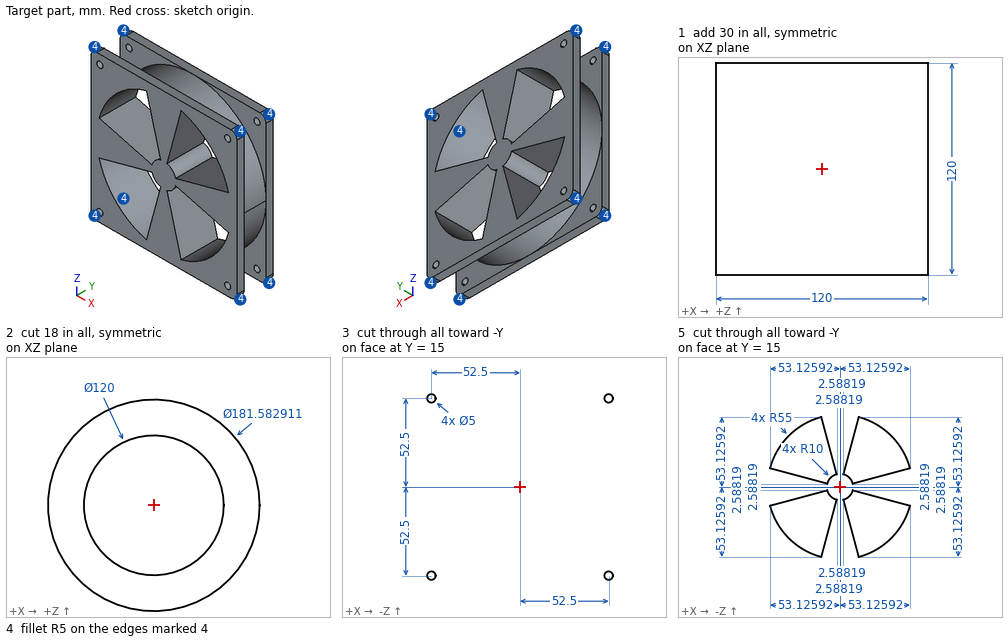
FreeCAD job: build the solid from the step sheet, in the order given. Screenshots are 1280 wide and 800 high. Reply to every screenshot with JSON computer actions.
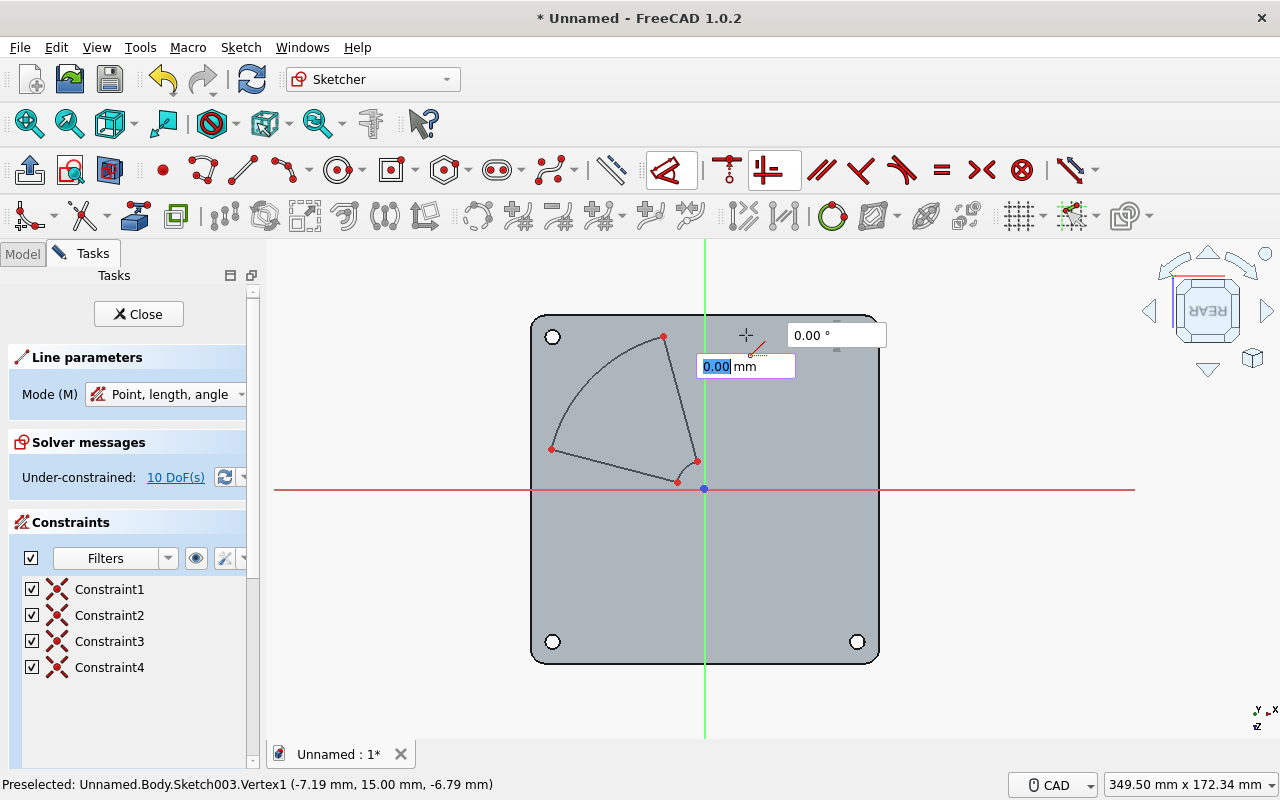
{"action": "scroll", "coordinate": [712, 462], "scroll_direction": "up", "scroll_amount": 4}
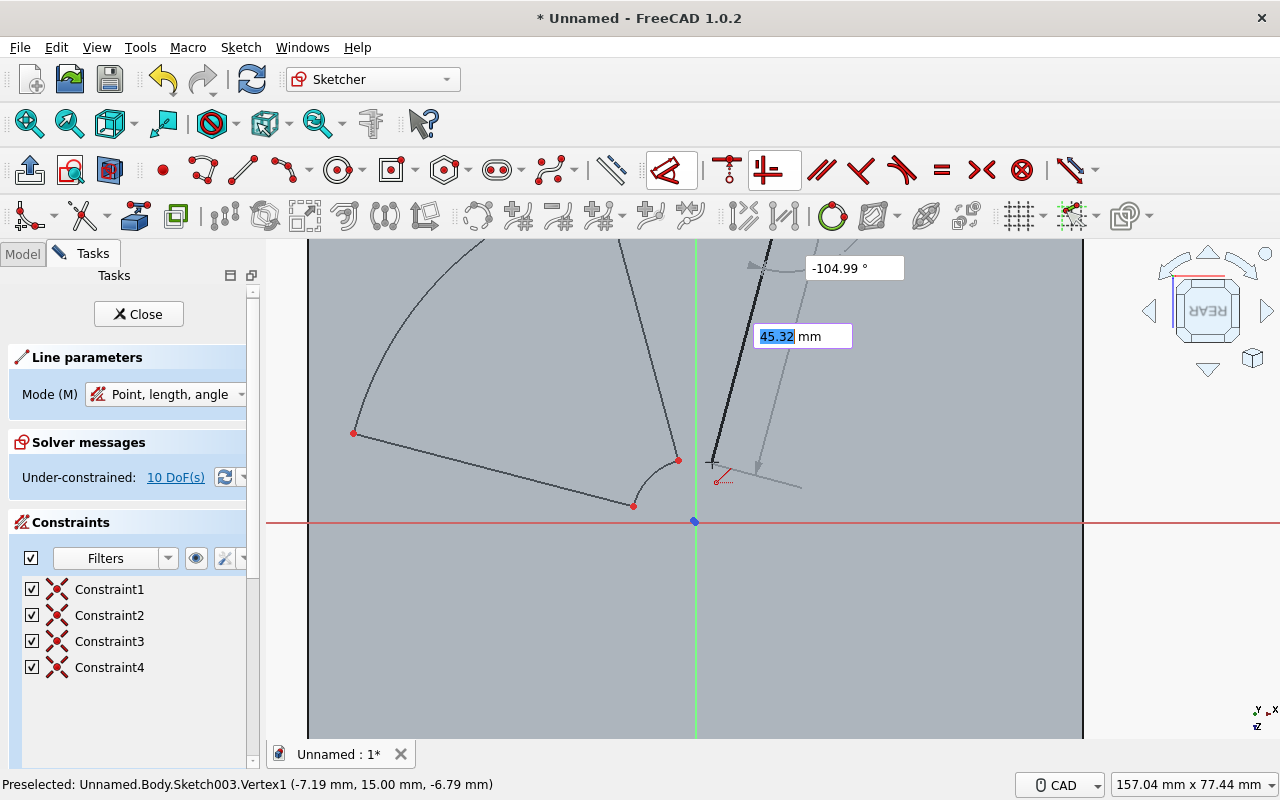
{"action": "left_click", "coordinate": [712, 460]}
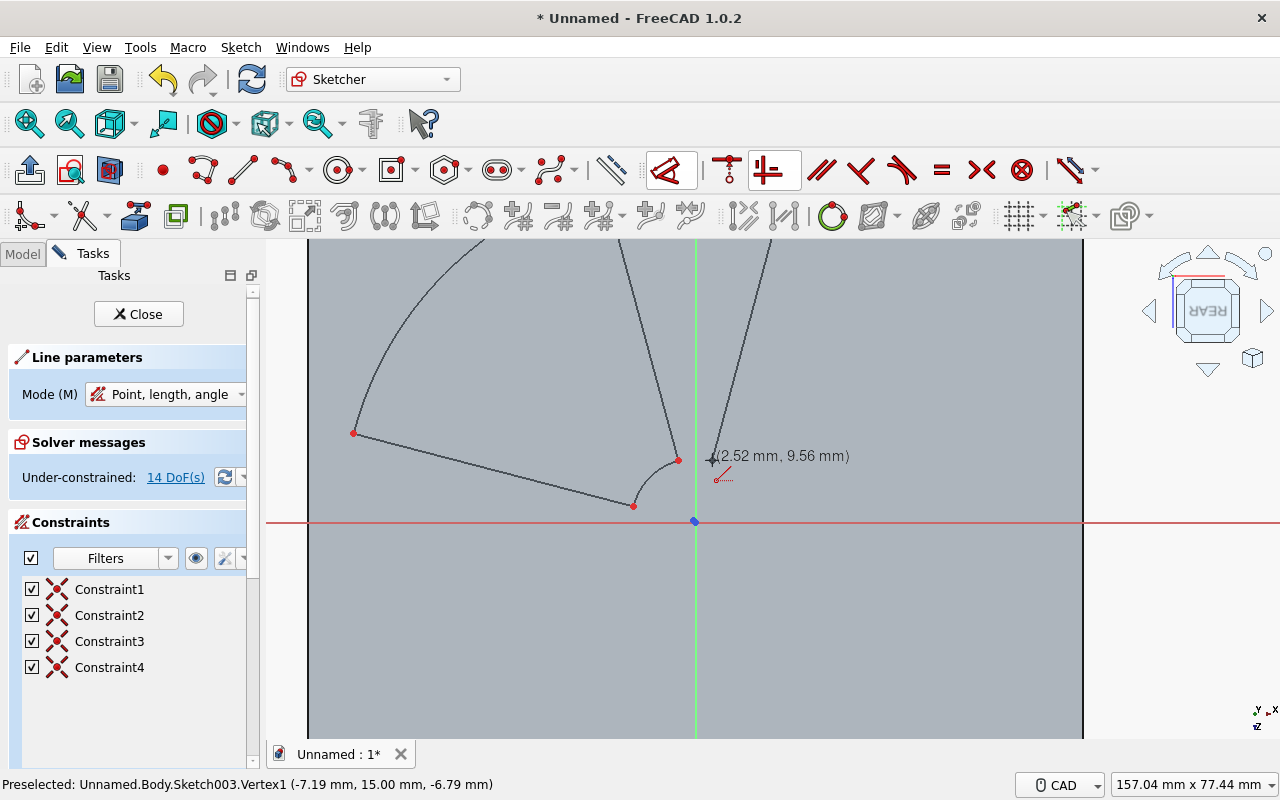
{"action": "left_click", "coordinate": [758, 506]}
{"action": "left_click", "coordinate": [1039, 431]}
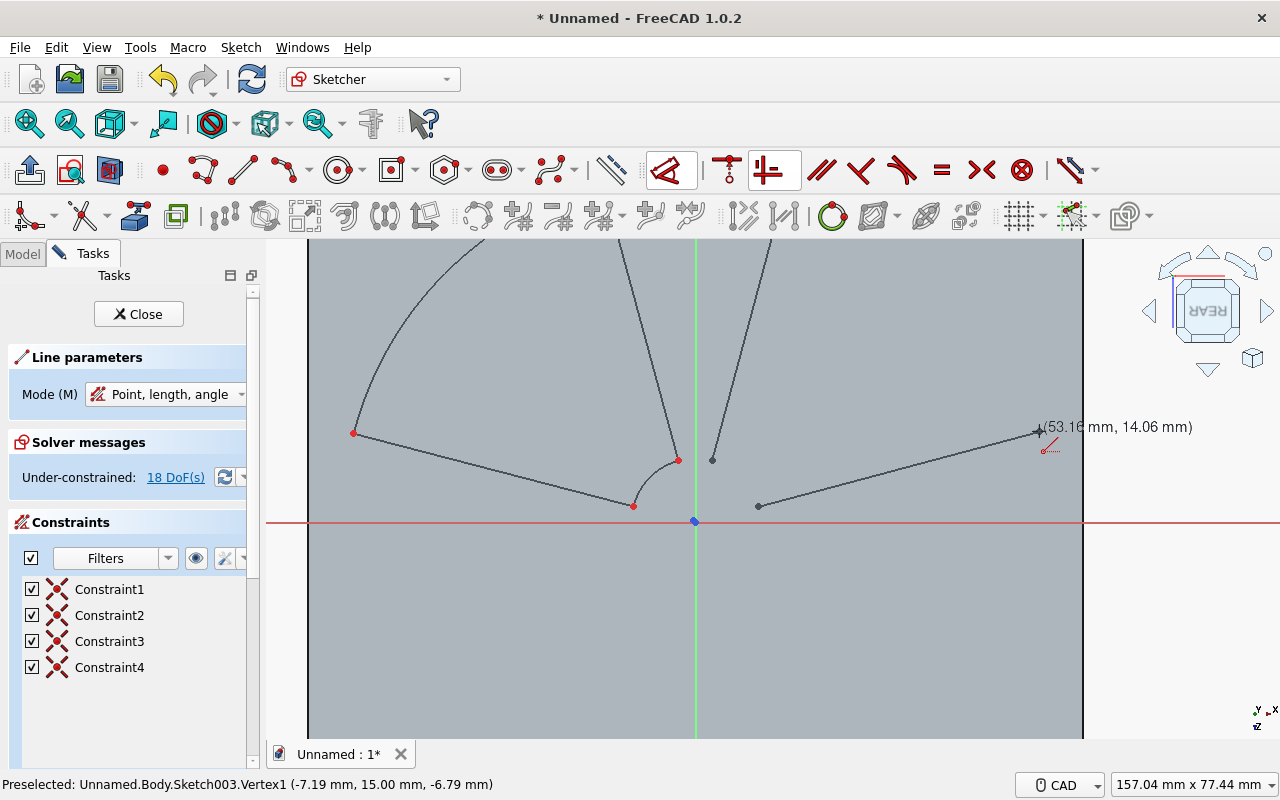
{"action": "left_click", "coordinate": [284, 170]}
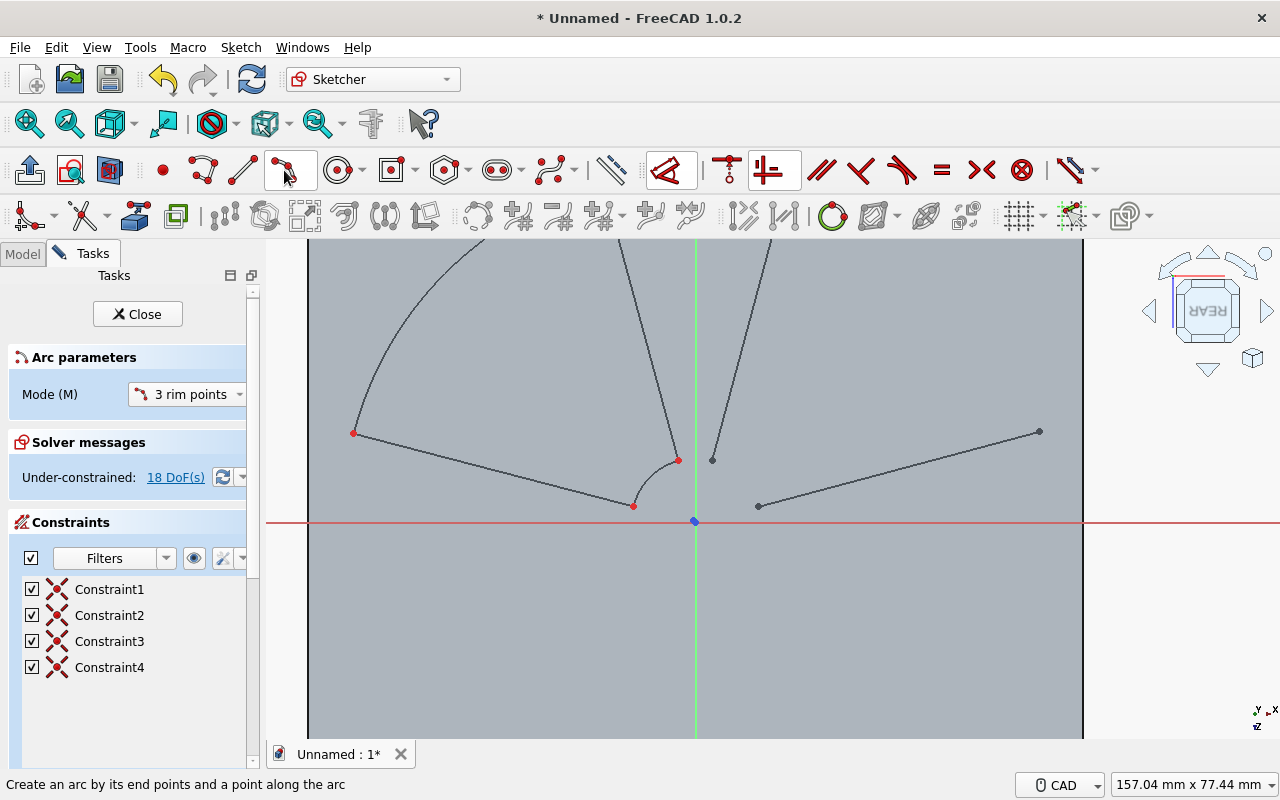
{"action": "left_click", "coordinate": [712, 461]}
{"action": "left_click", "coordinate": [758, 507]}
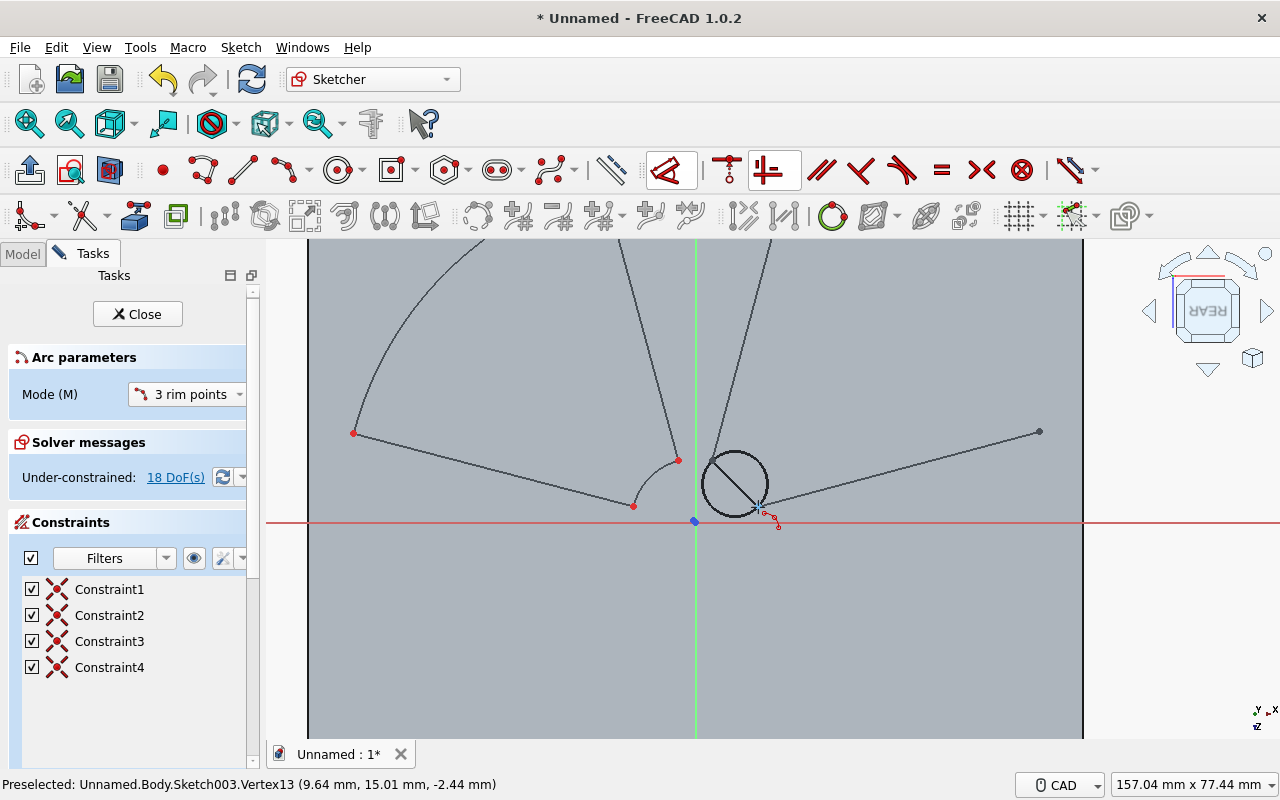
{"action": "scroll", "coordinate": [741, 477], "scroll_direction": "up", "scroll_amount": 4}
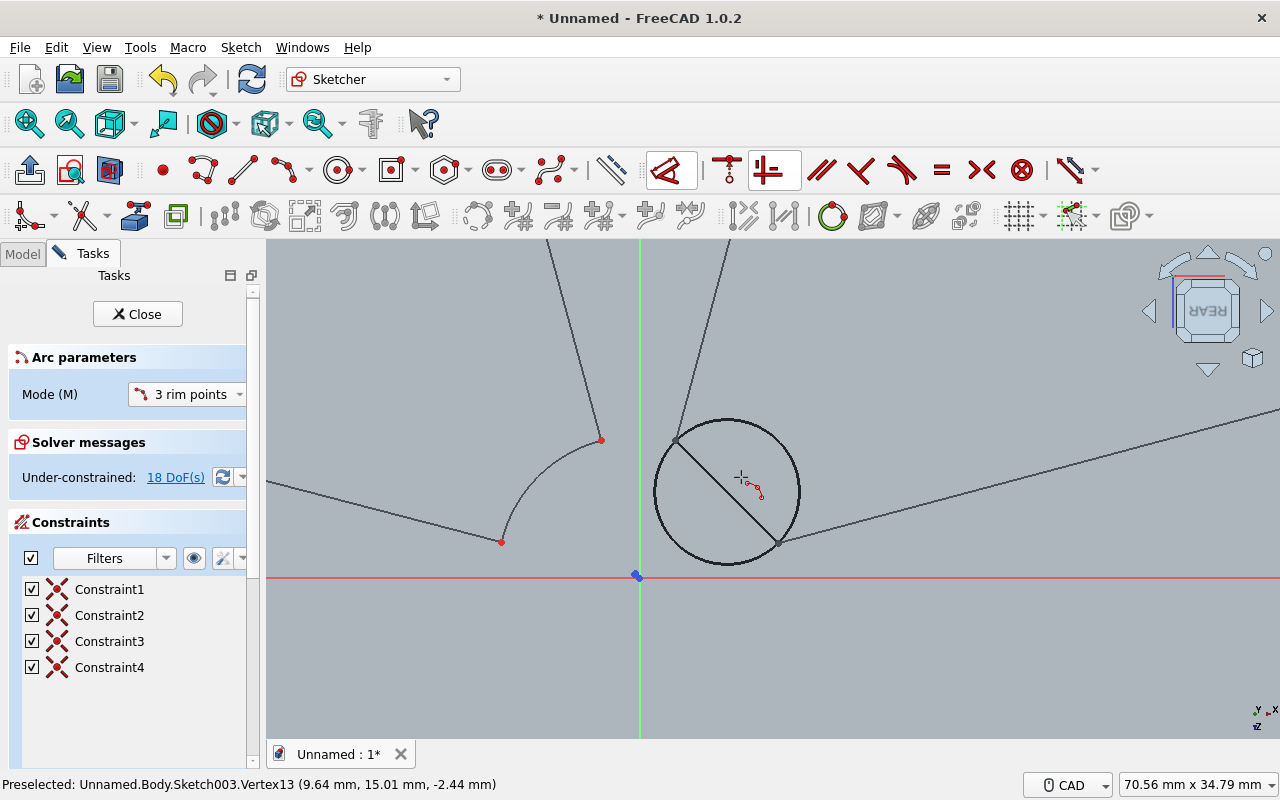
{"action": "left_click", "coordinate": [741, 477]}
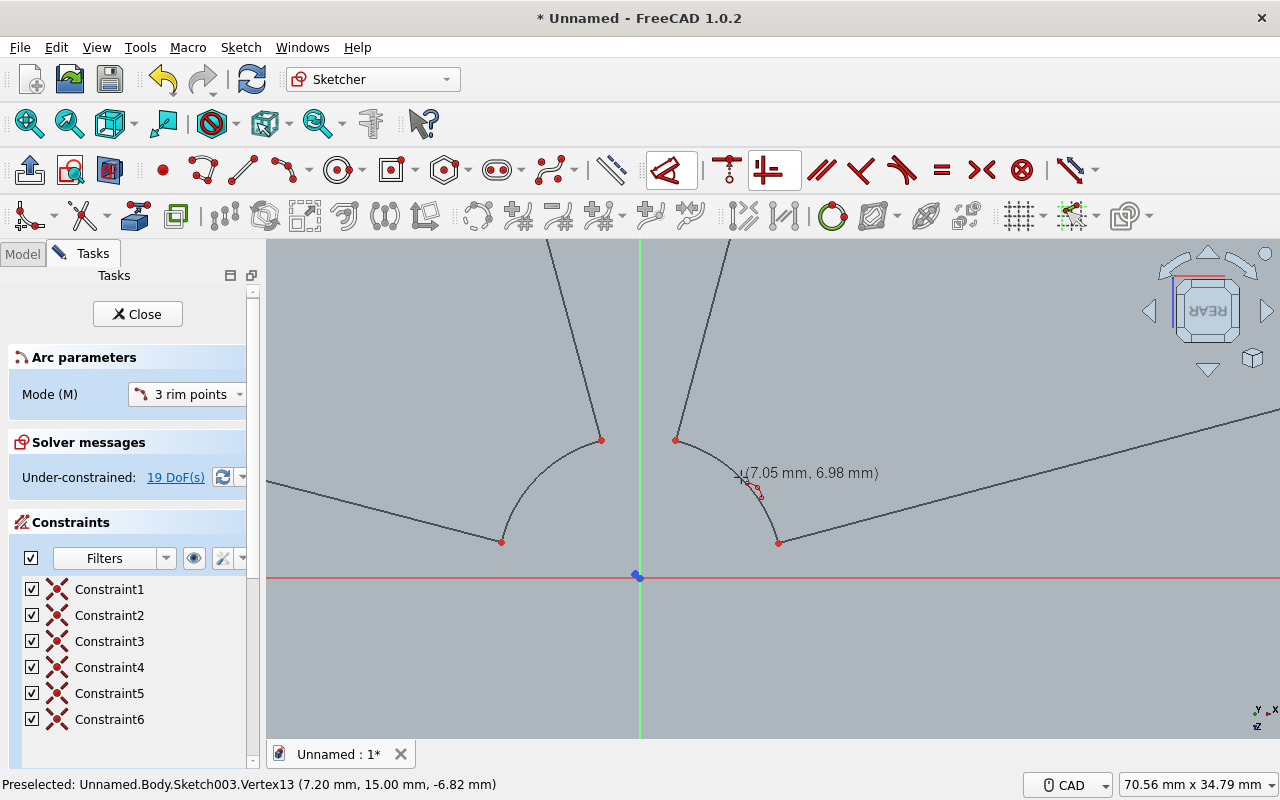
{"action": "scroll", "coordinate": [721, 466], "scroll_direction": "down", "scroll_amount": 8}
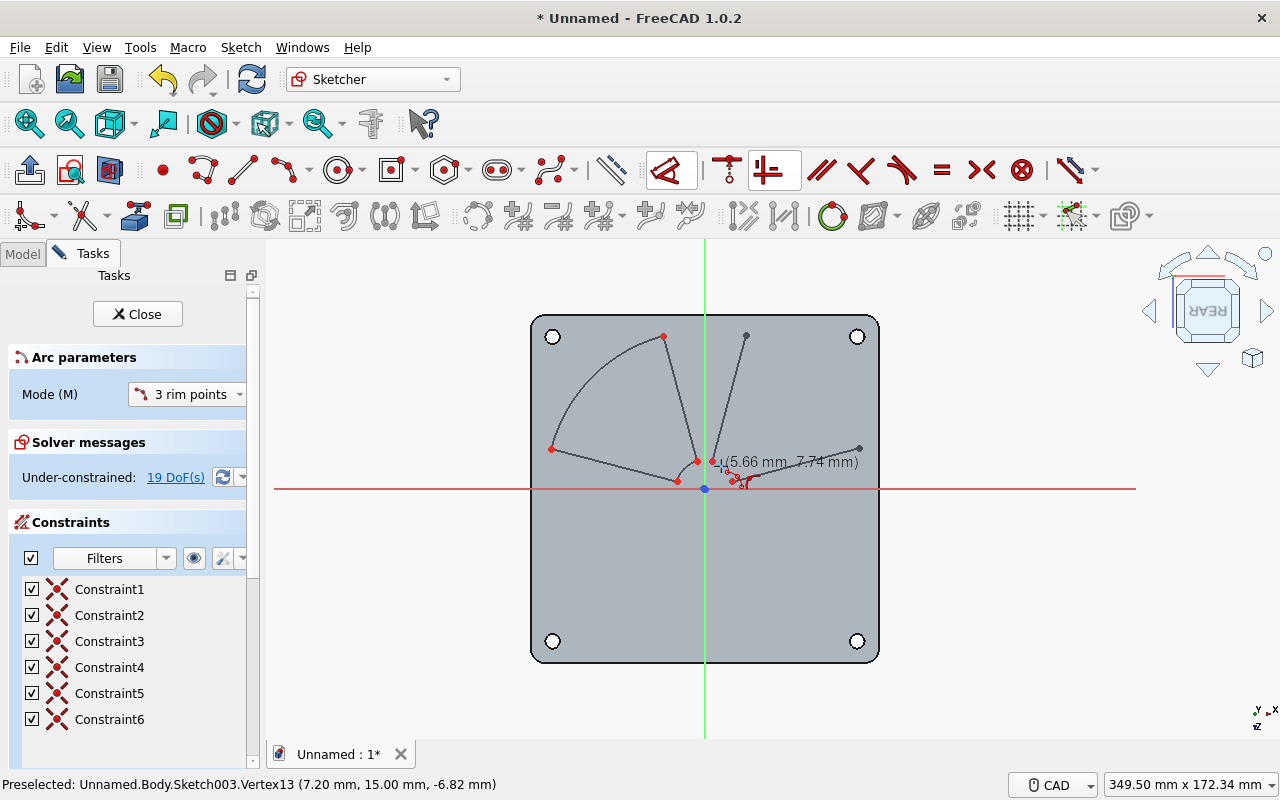
{"action": "left_click", "coordinate": [859, 448]}
{"action": "left_click", "coordinate": [746, 335]}
{"action": "left_click", "coordinate": [818, 376]}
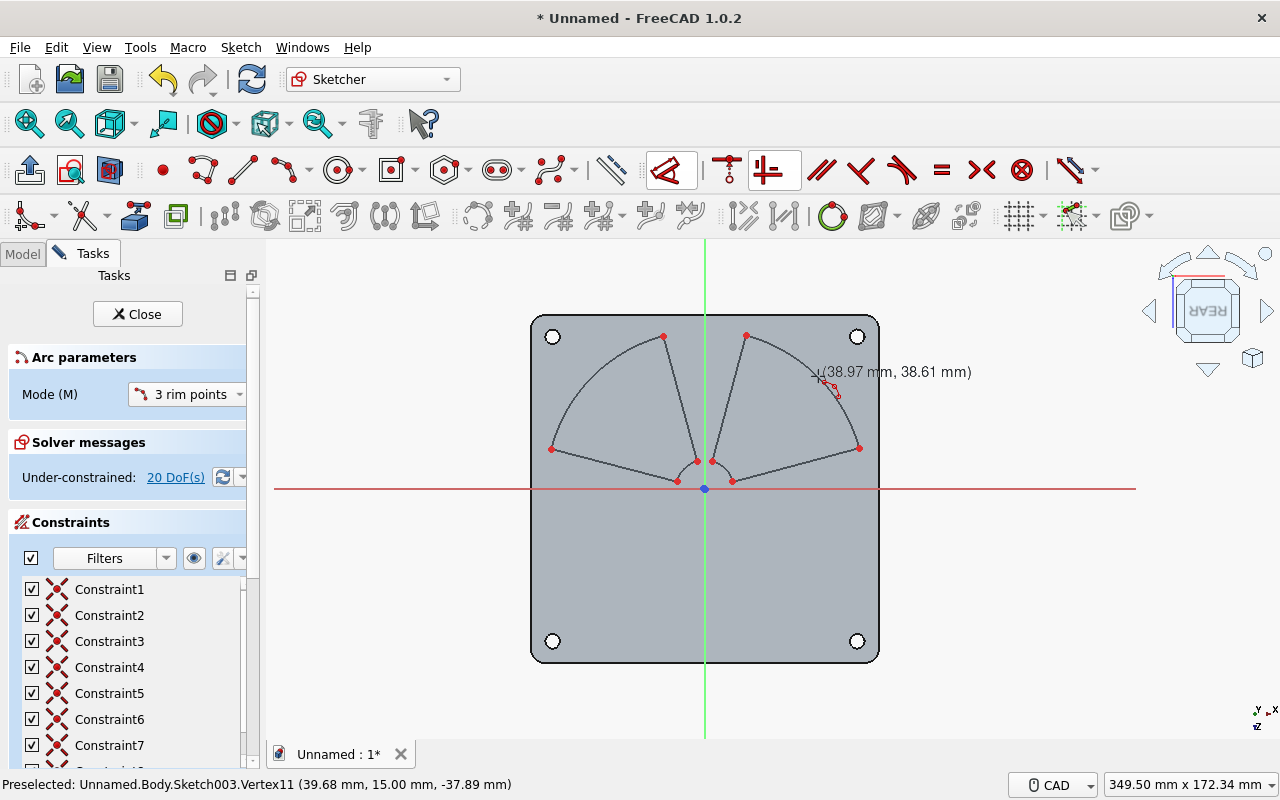
{"action": "left_click", "coordinate": [244, 170]}